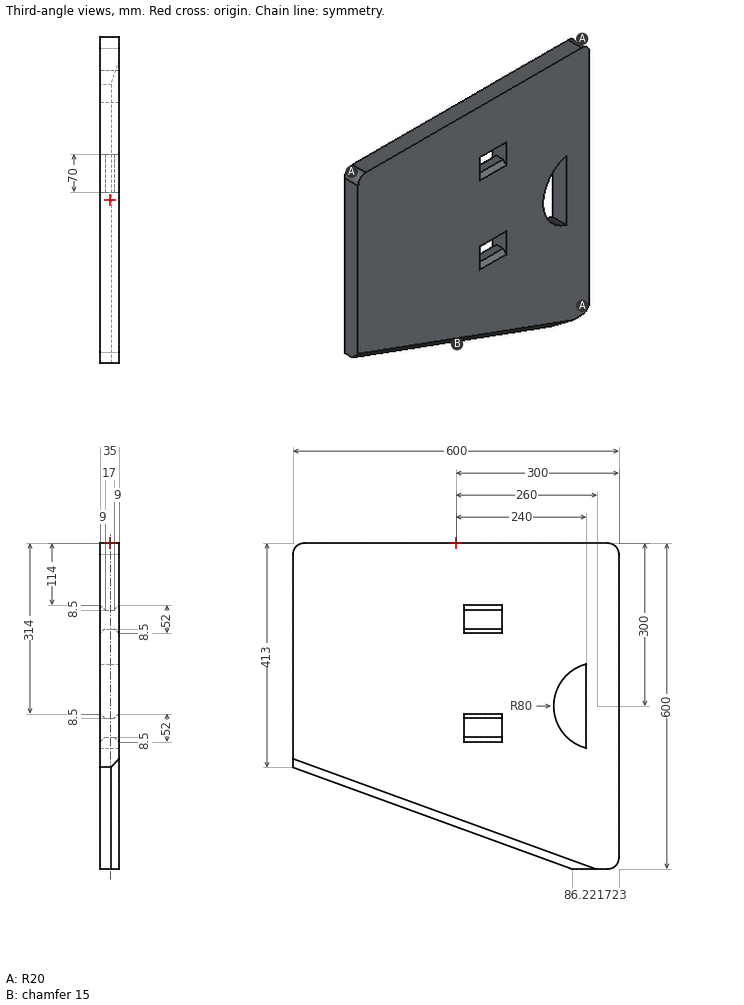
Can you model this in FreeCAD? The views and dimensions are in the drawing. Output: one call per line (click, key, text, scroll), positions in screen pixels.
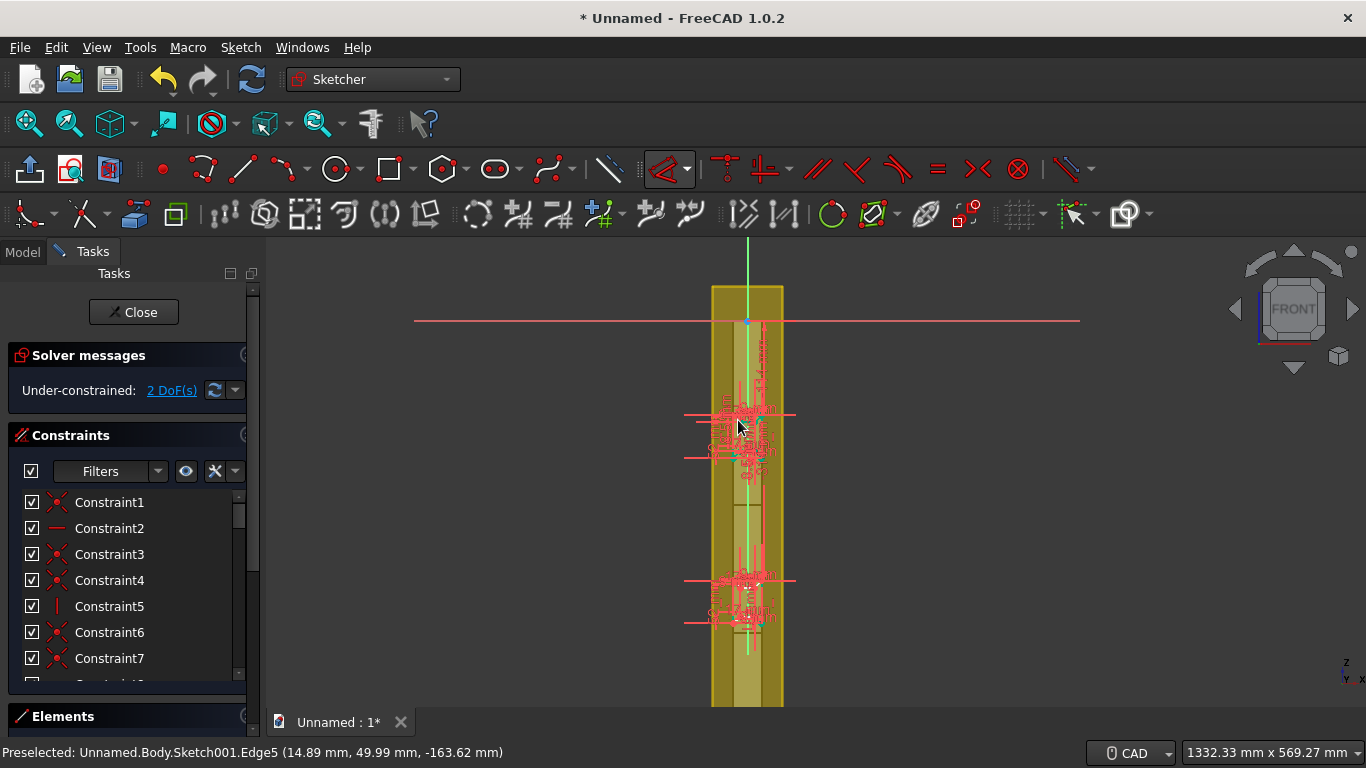
scroll(735, 583, up, 10)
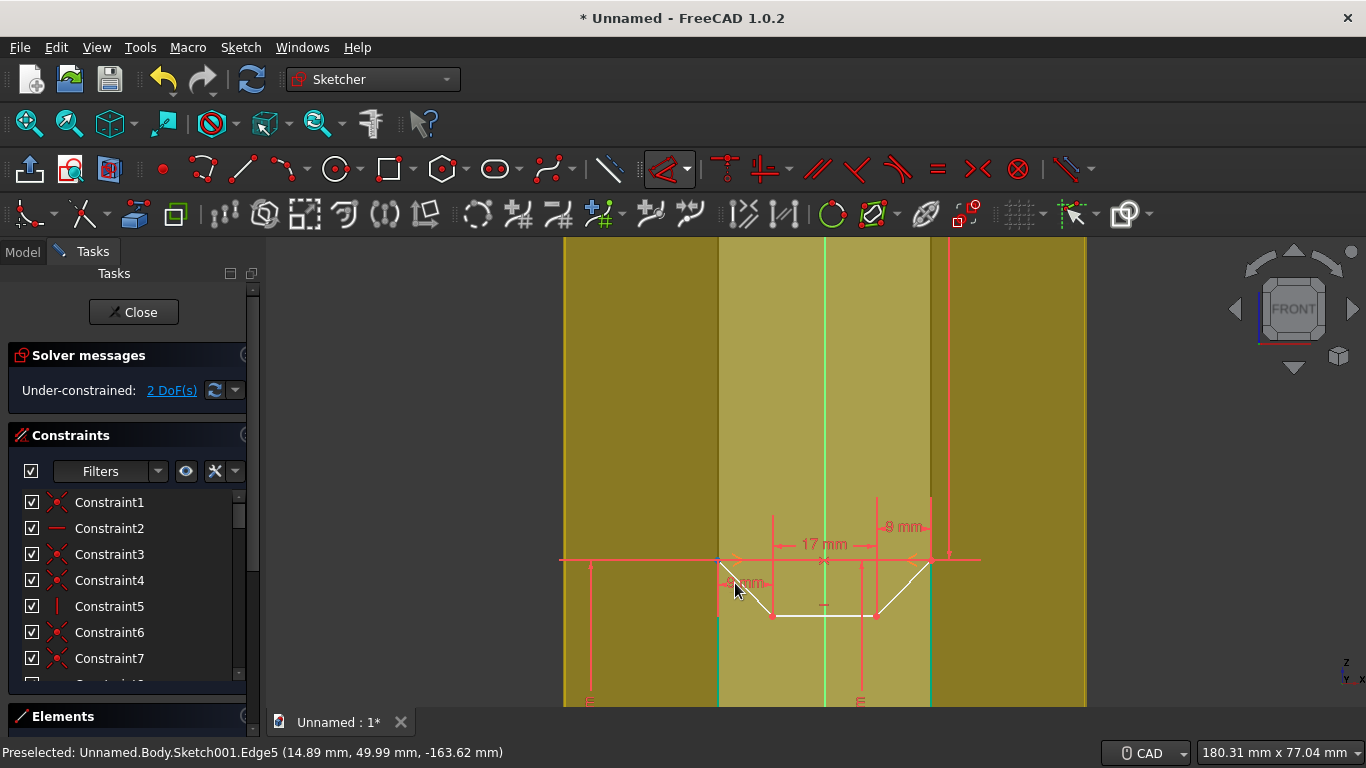
click(756, 599)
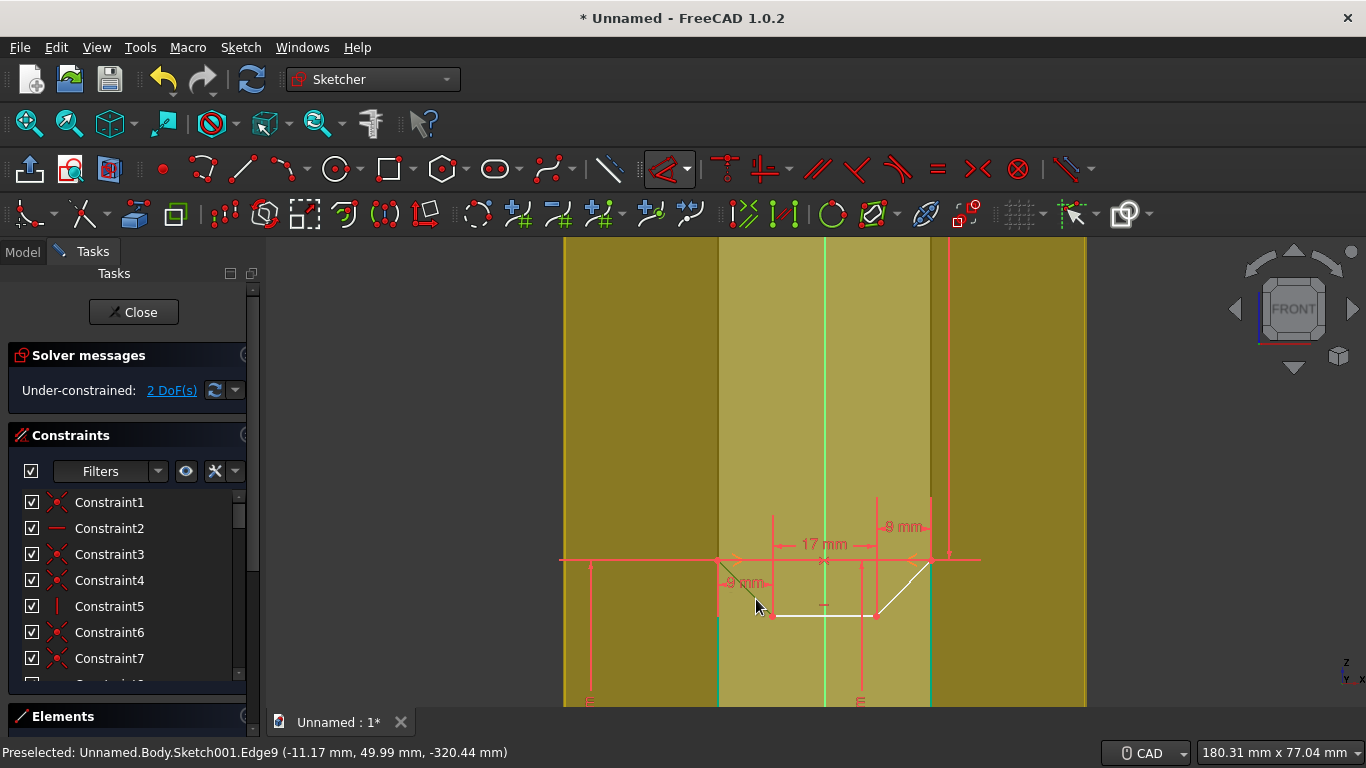
key(i)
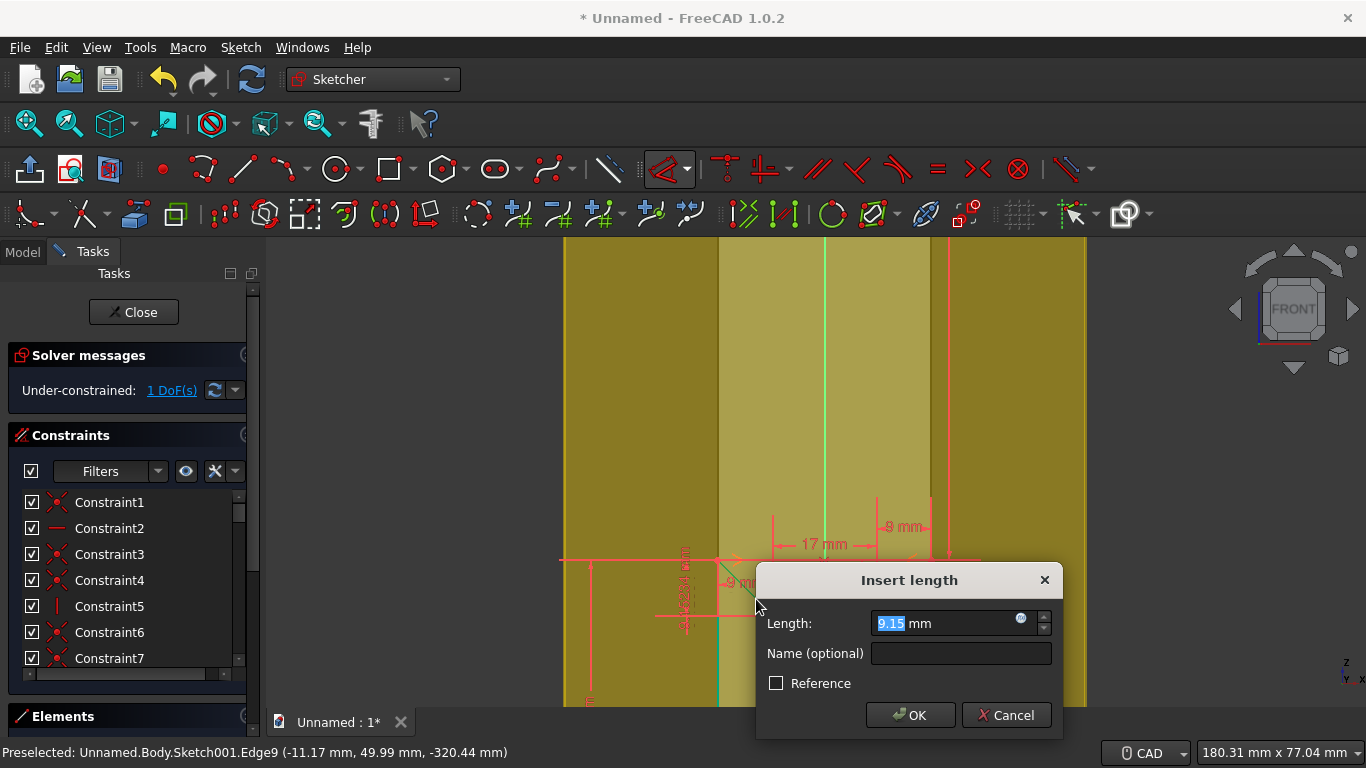
text(8.5)
key(Return)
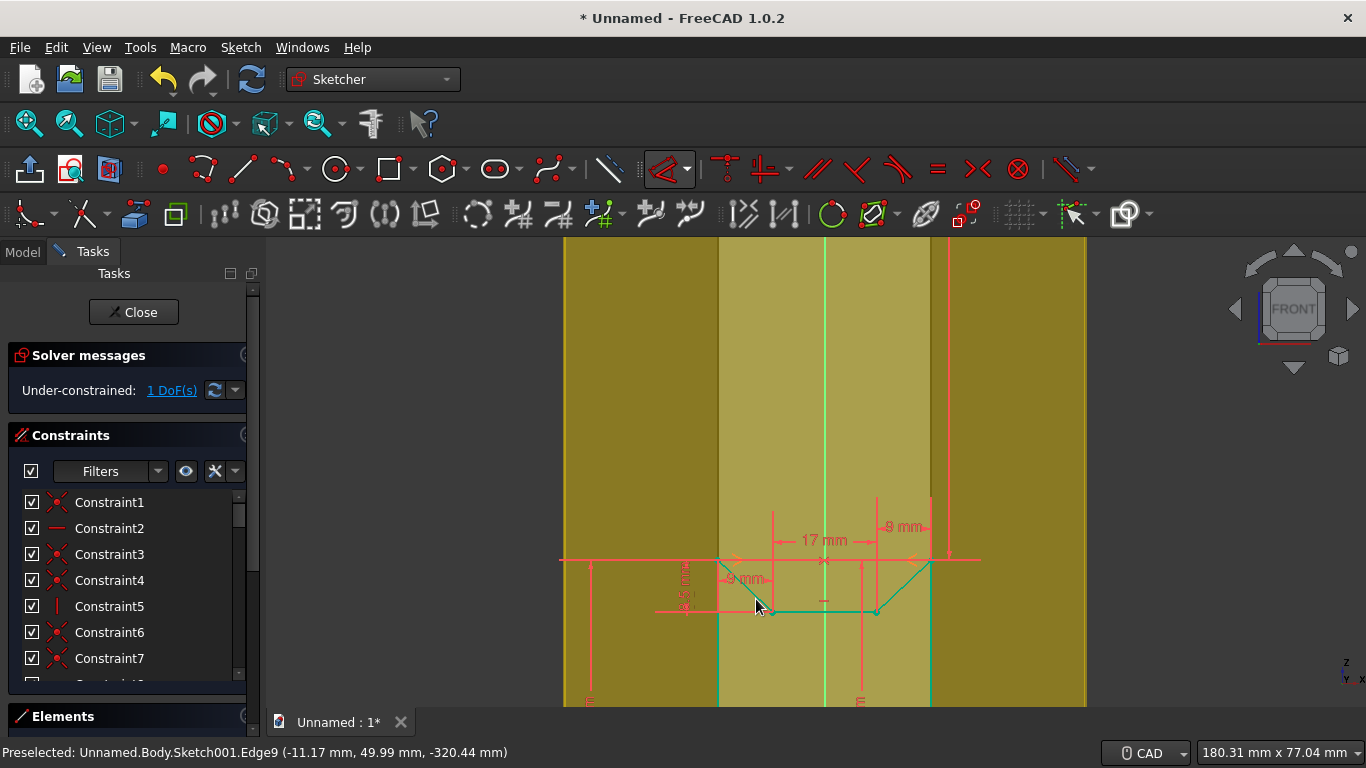
scroll(735, 583, down, 10)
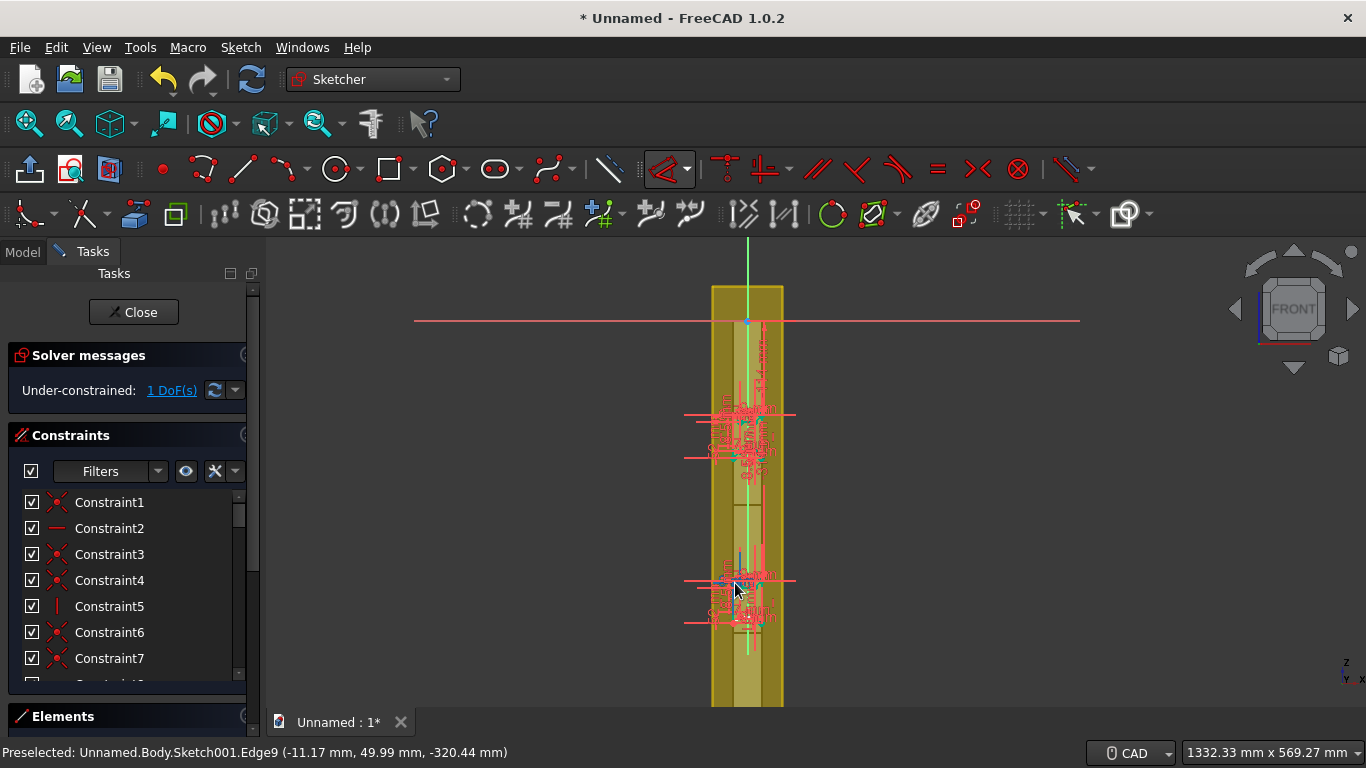
scroll(760, 622, up, 10)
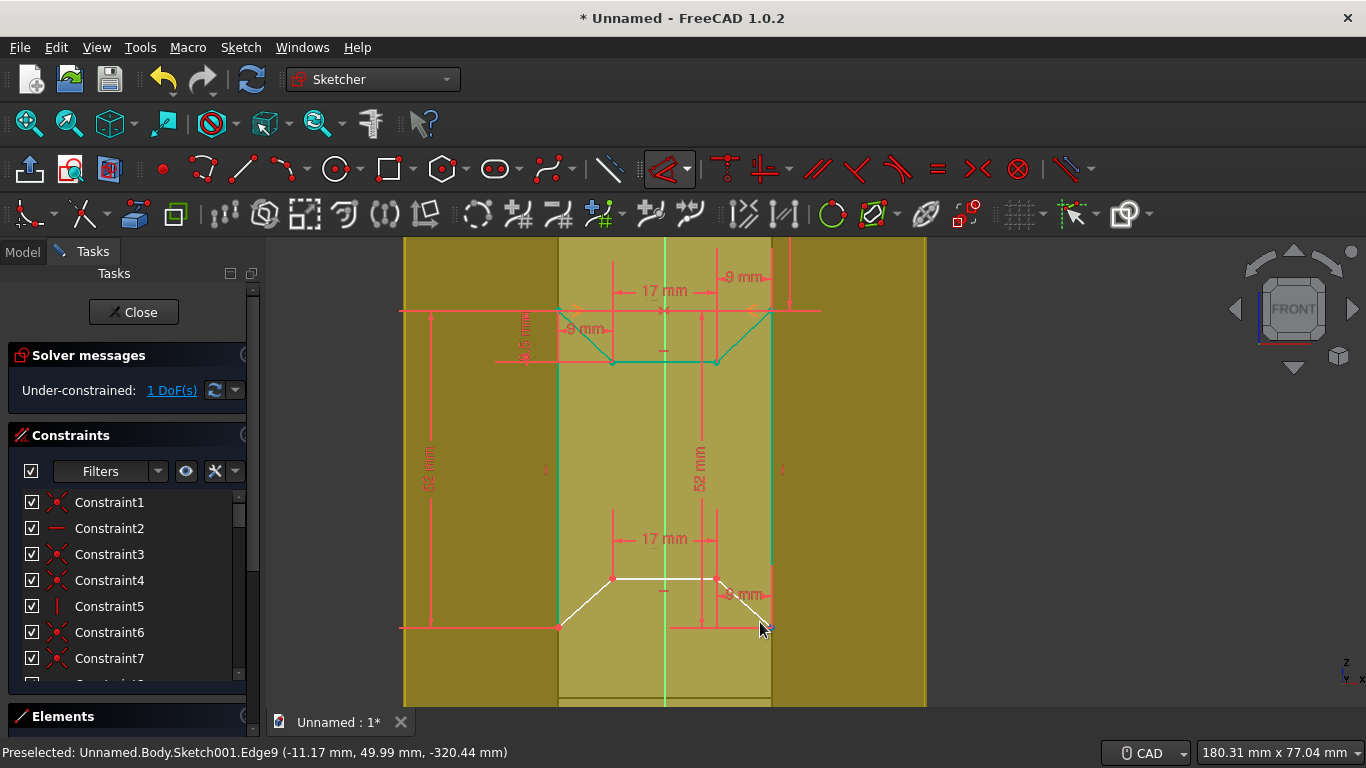
click(755, 613)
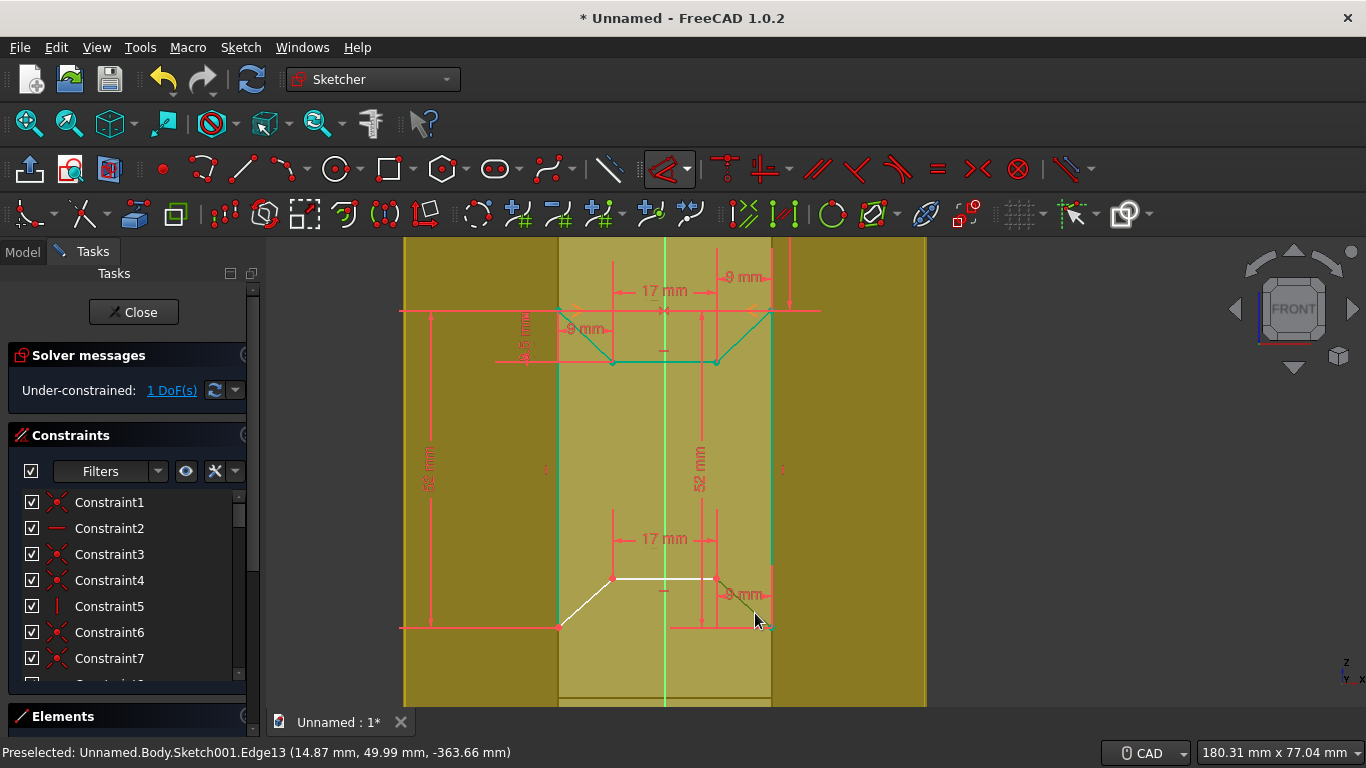
click(690, 170)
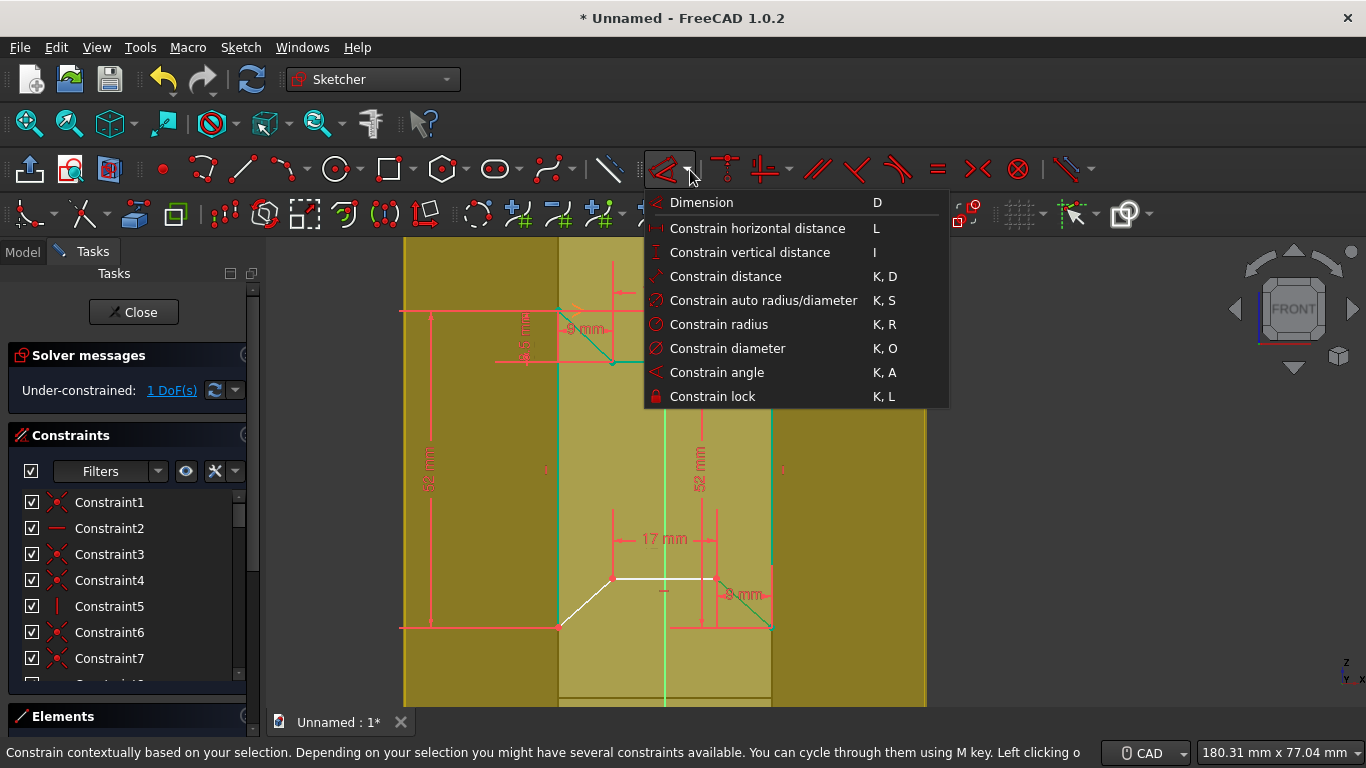
click(797, 252)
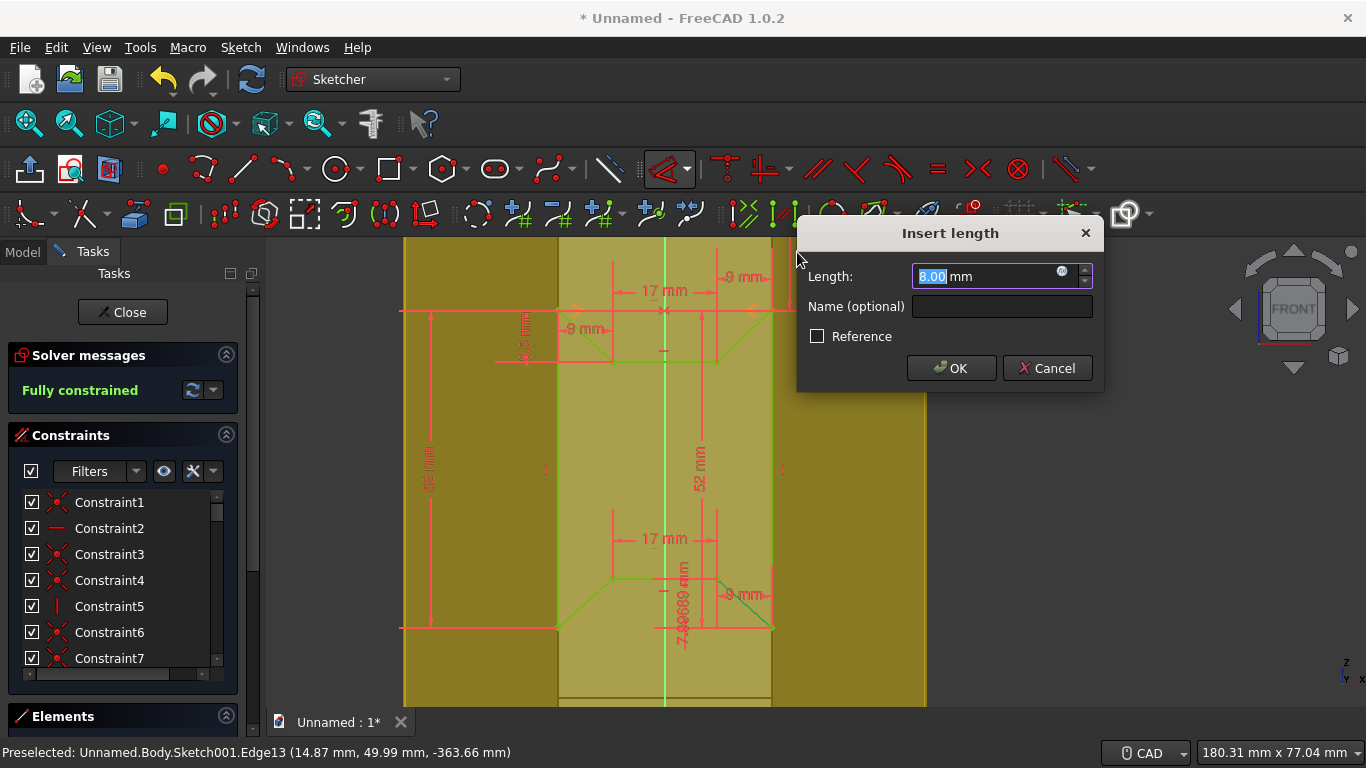
text(8.5)
key(Return)